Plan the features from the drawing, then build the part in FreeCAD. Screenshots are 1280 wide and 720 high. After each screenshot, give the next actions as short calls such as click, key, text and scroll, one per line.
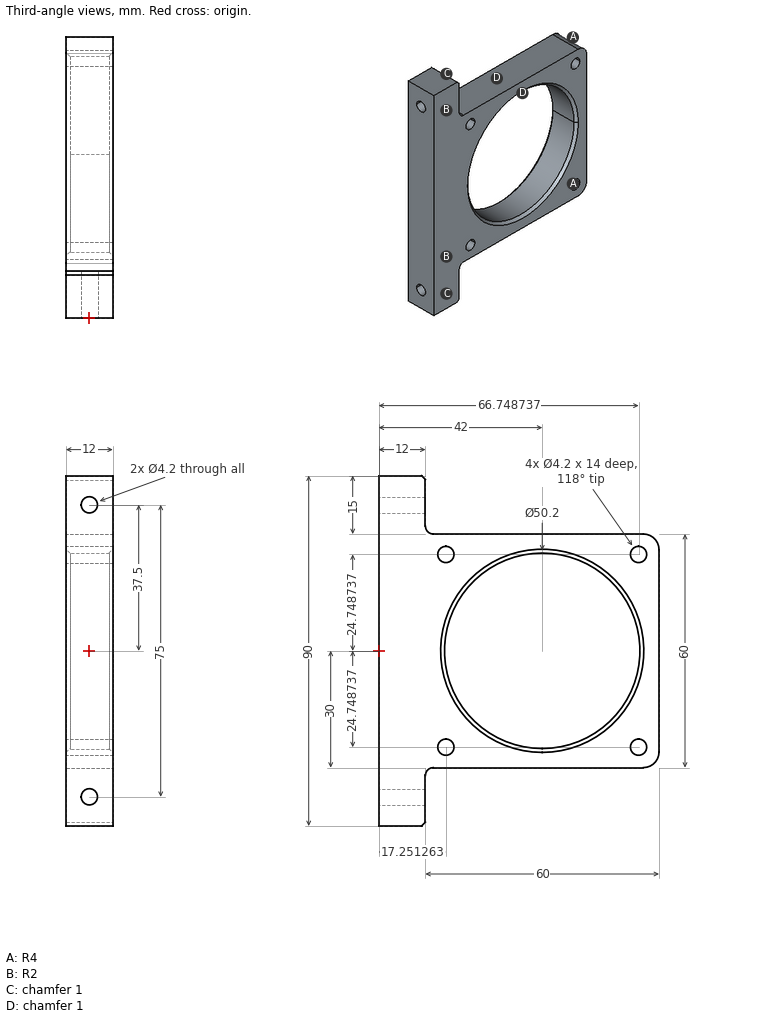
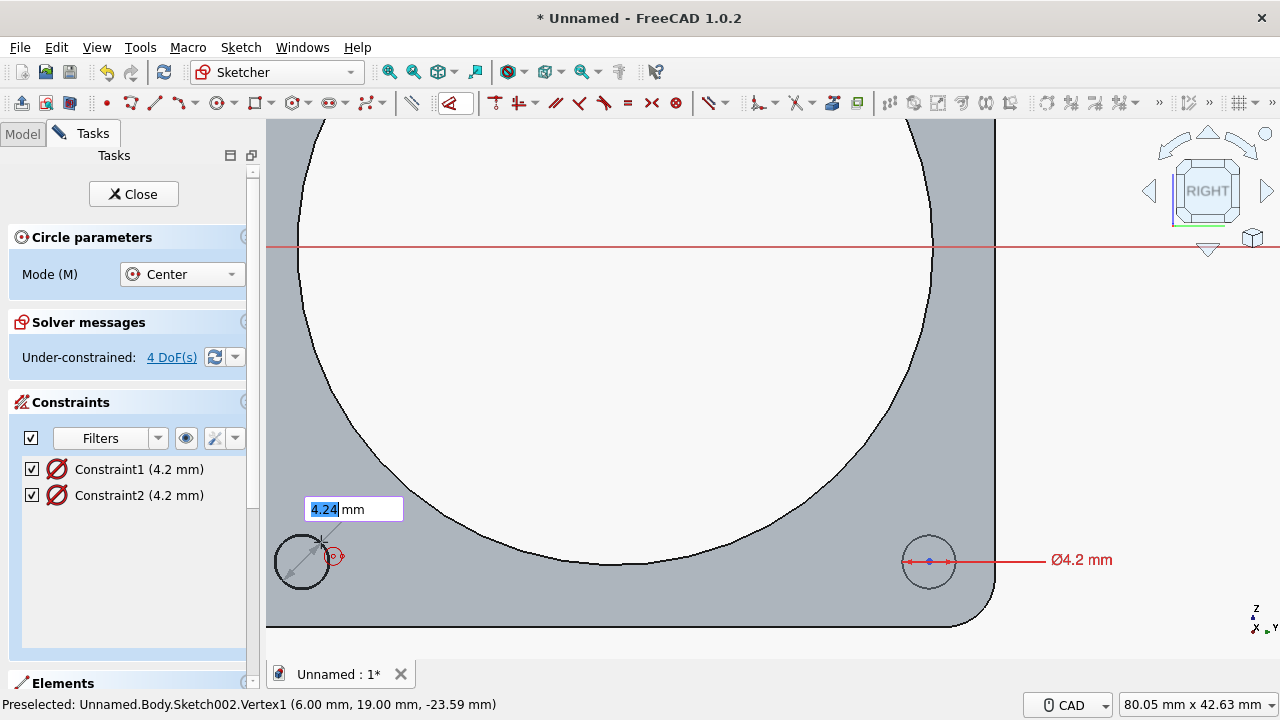
text(4.2)
key(Return)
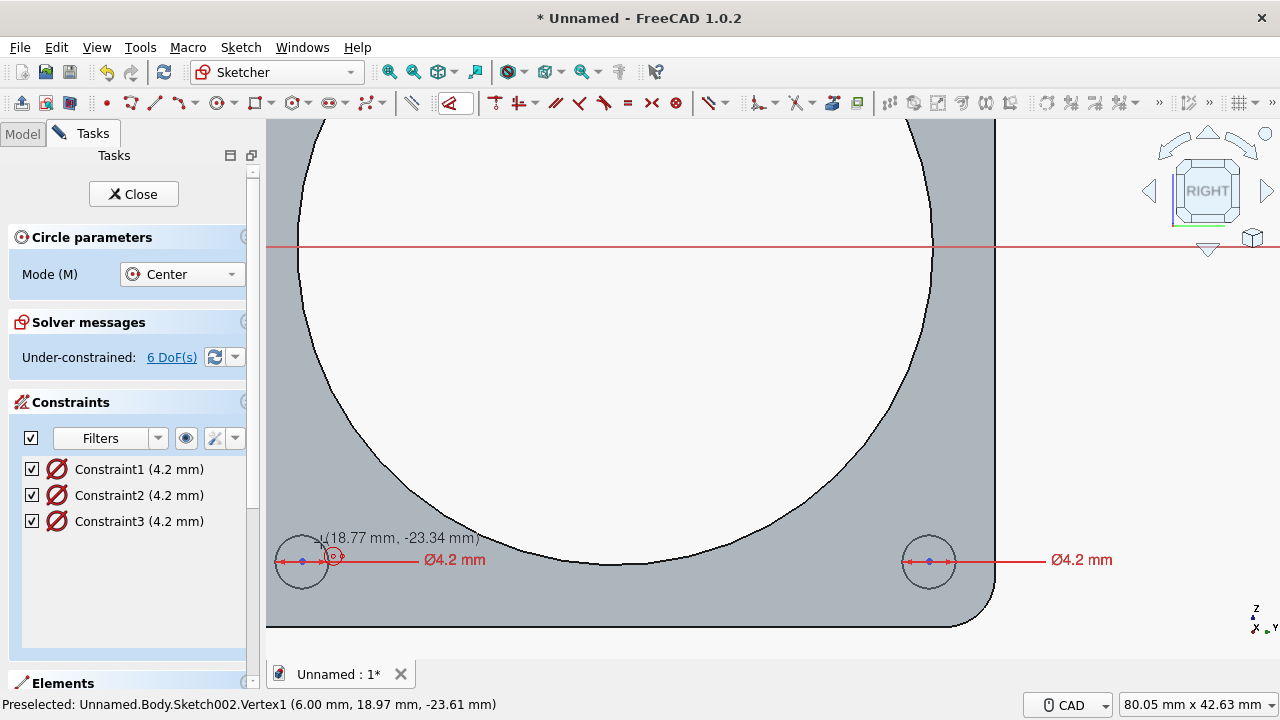
scroll(930, 561, down, 3)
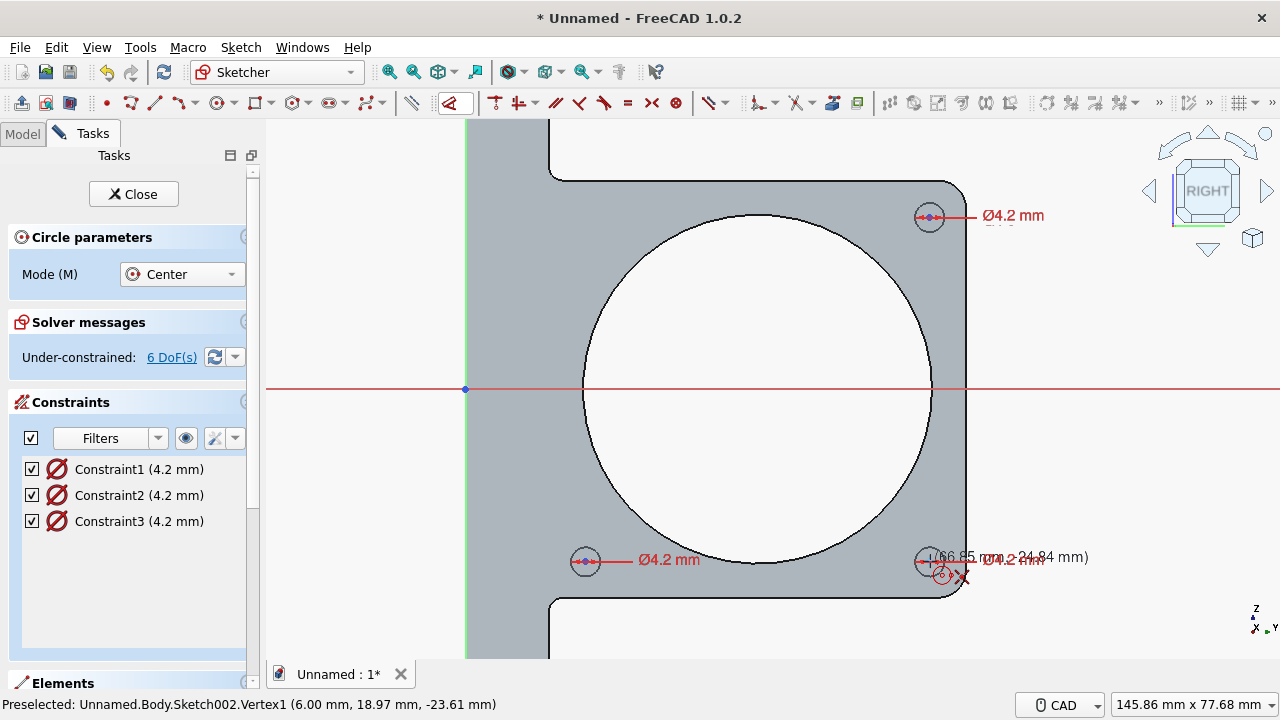
scroll(585, 217, up, 3)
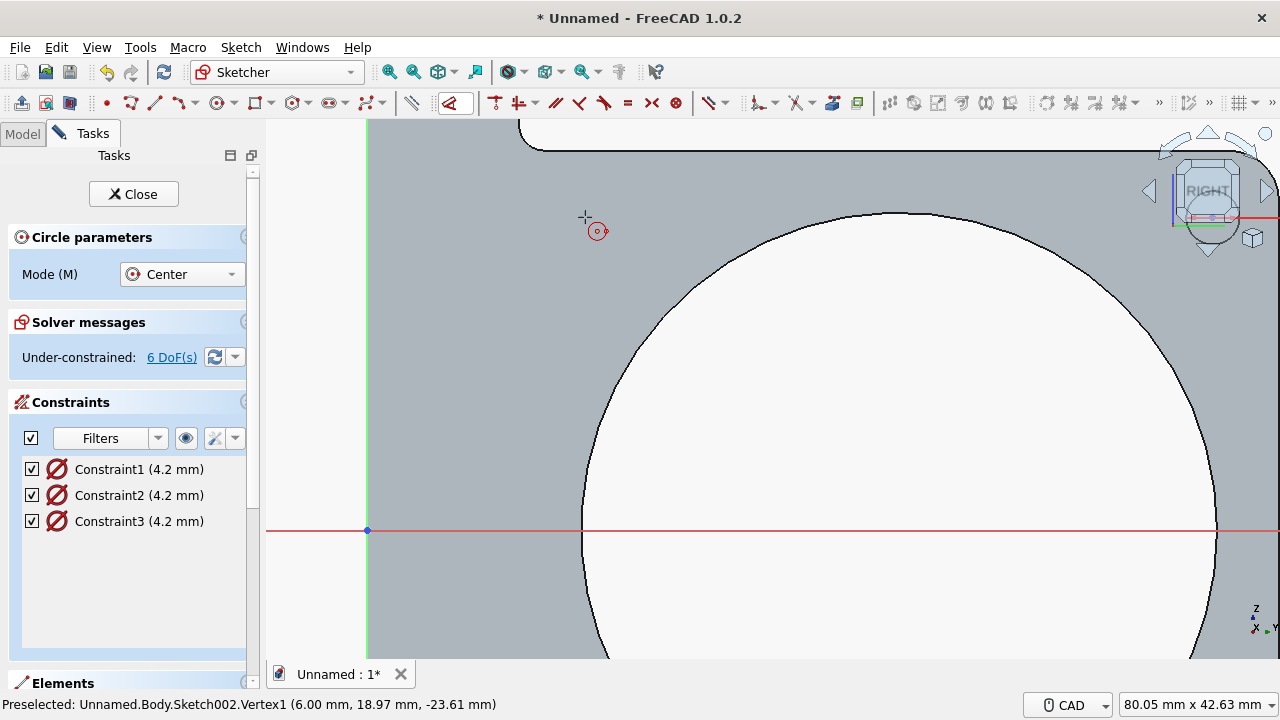
click(586, 217)
move(604, 198)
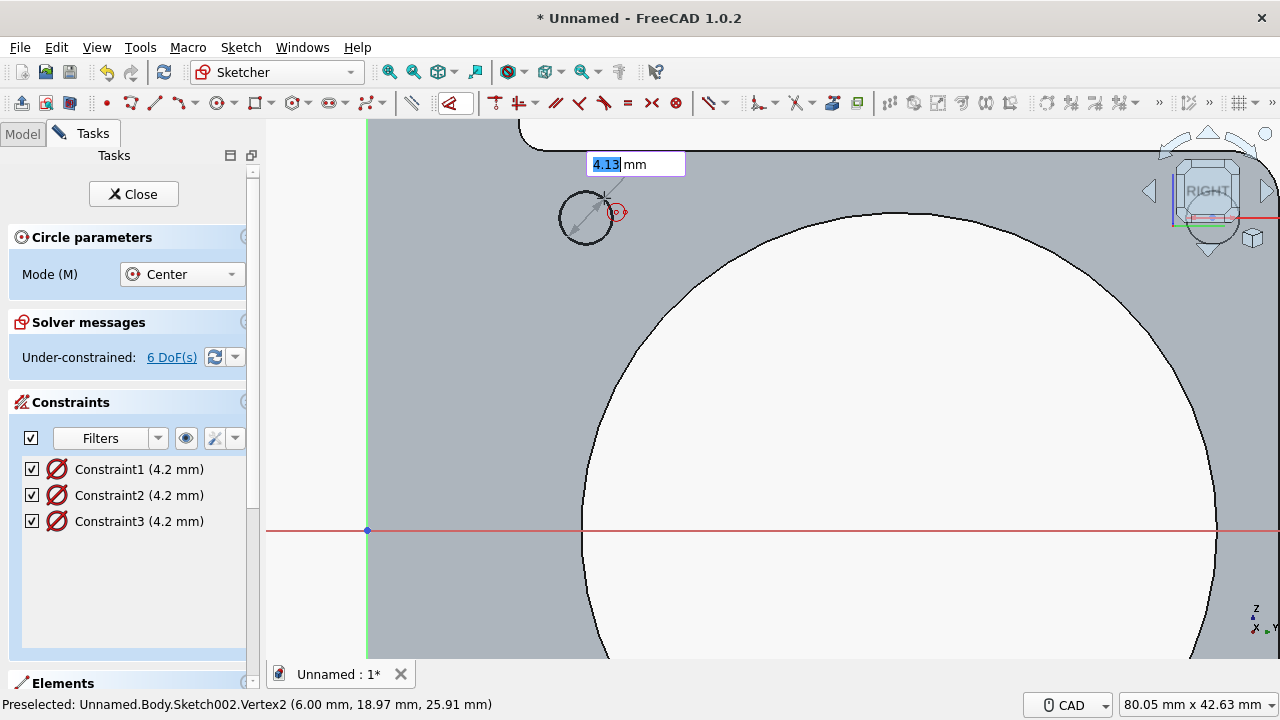
text(4.2)
key(Return)
key(Escape)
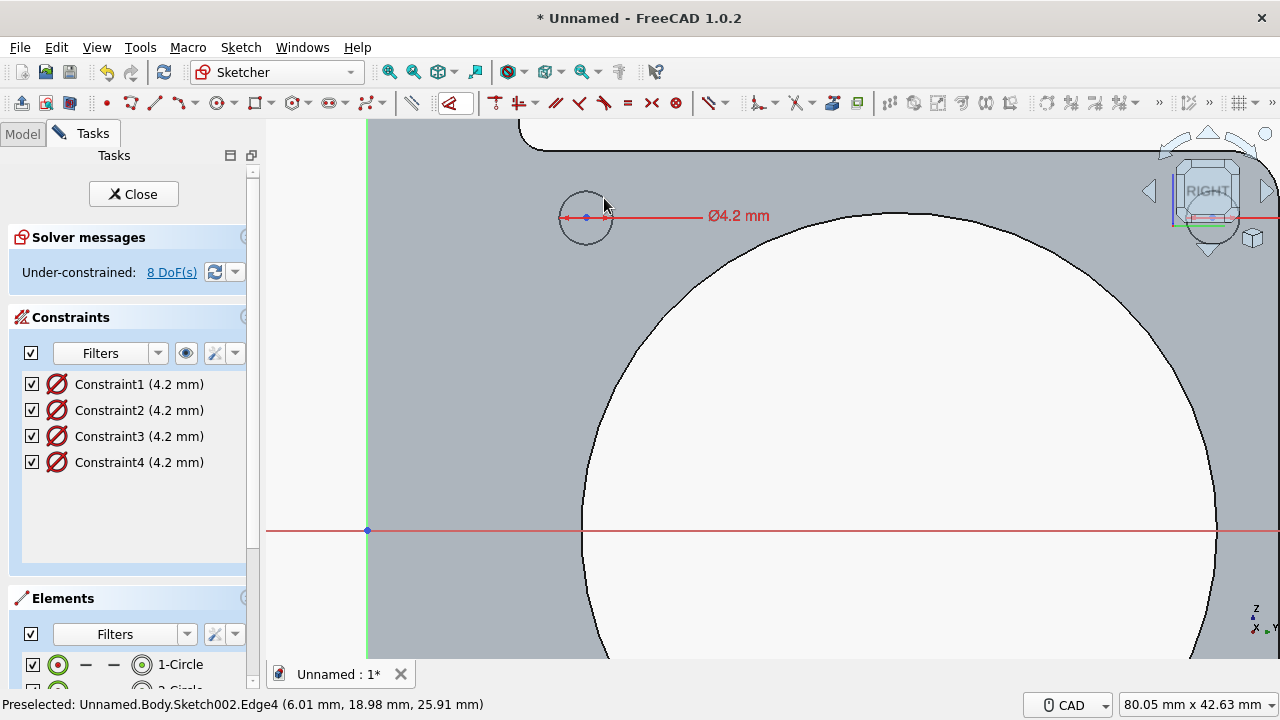
scroll(585, 217, down, 3)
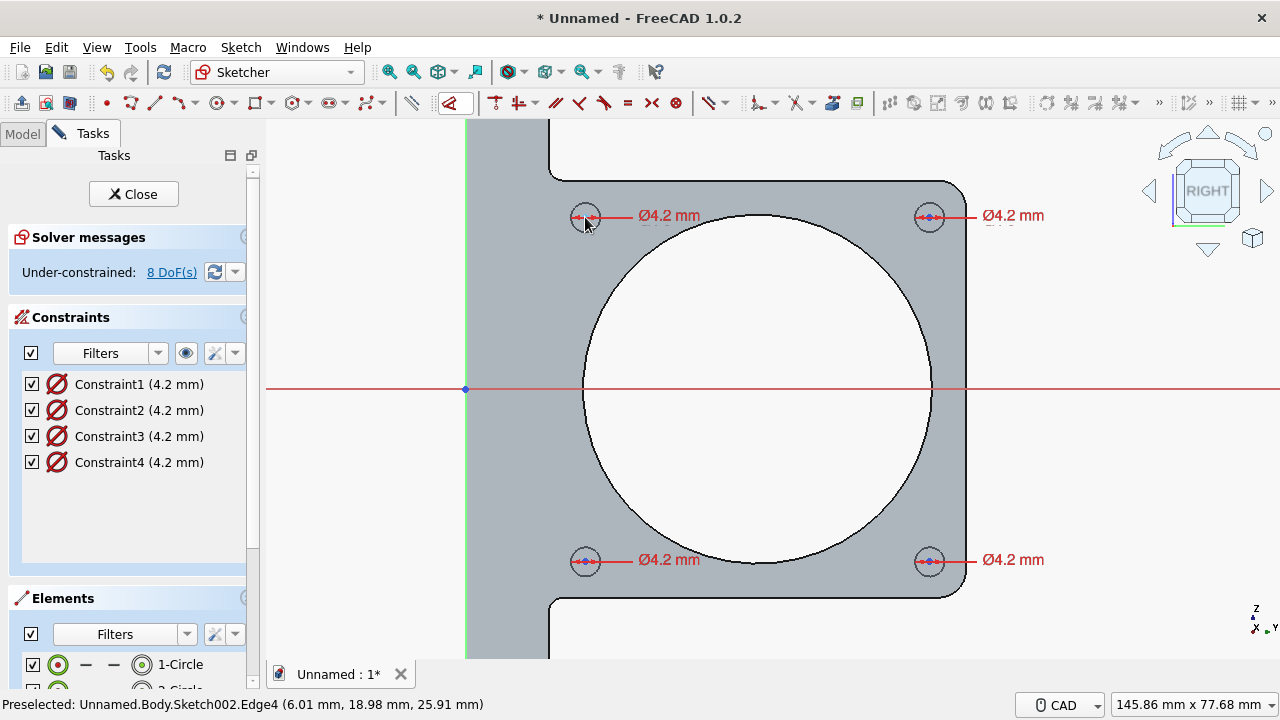
click(930, 218)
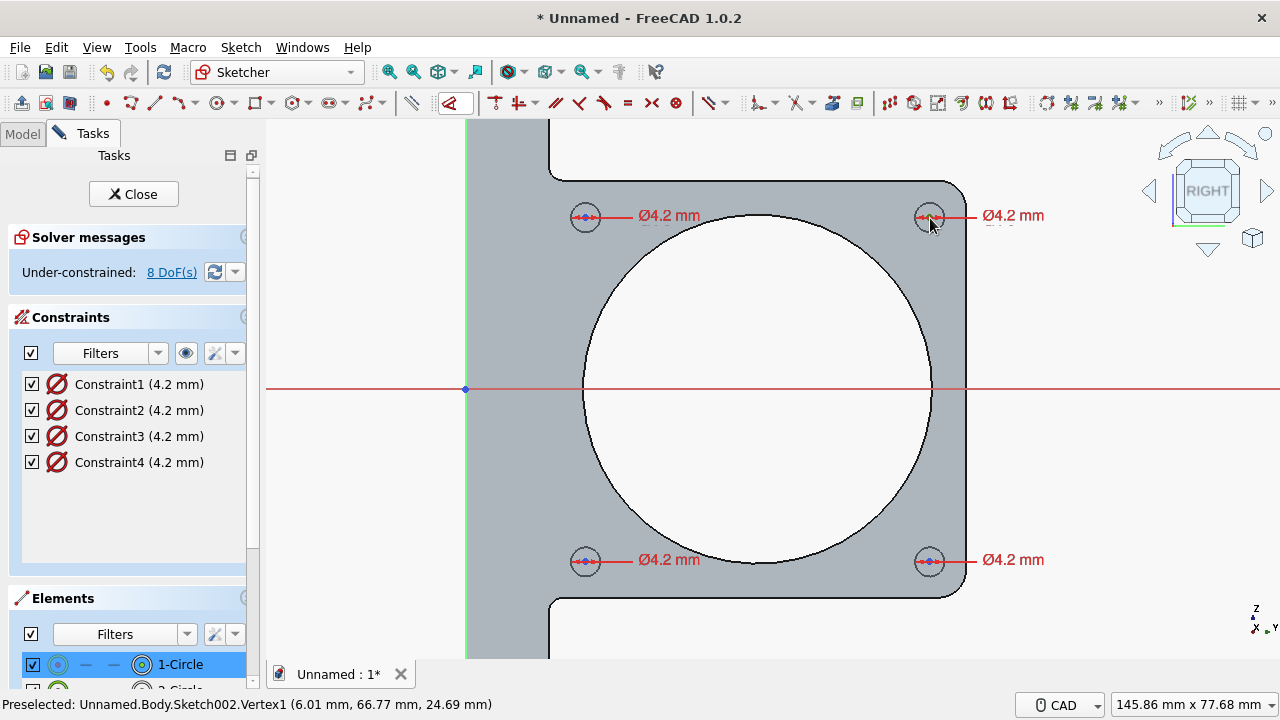
click(930, 562)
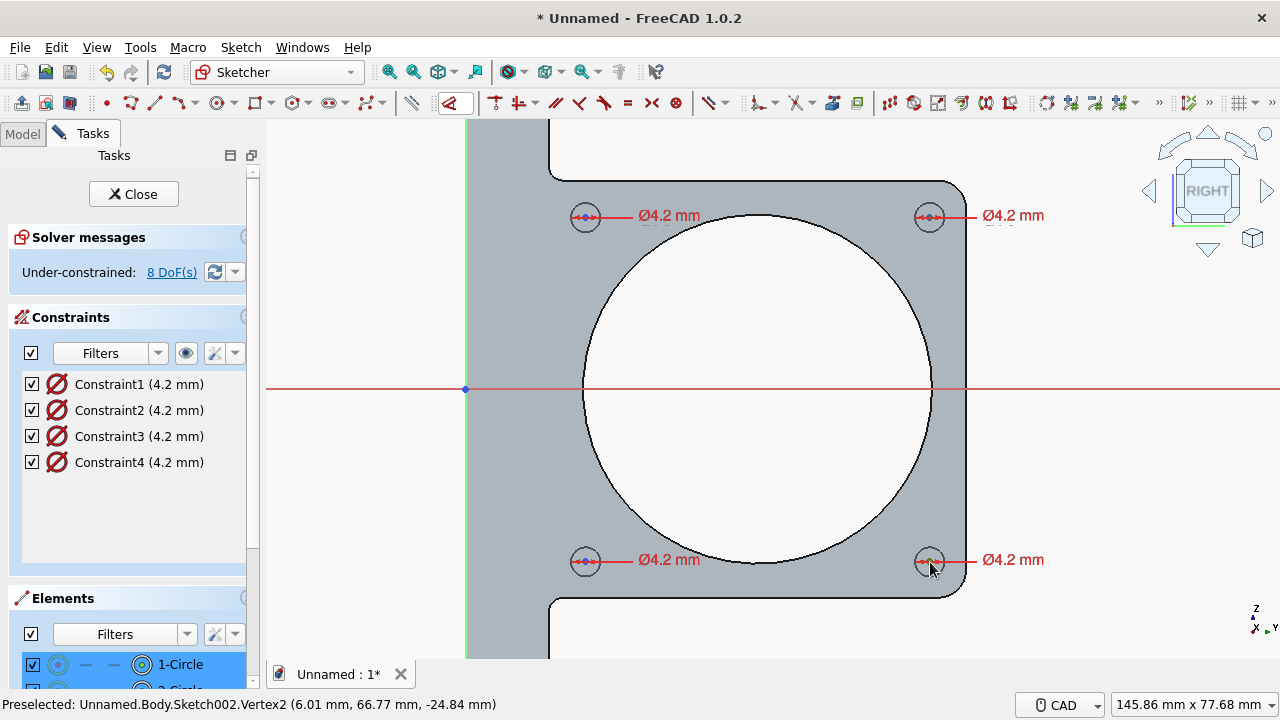
key(v)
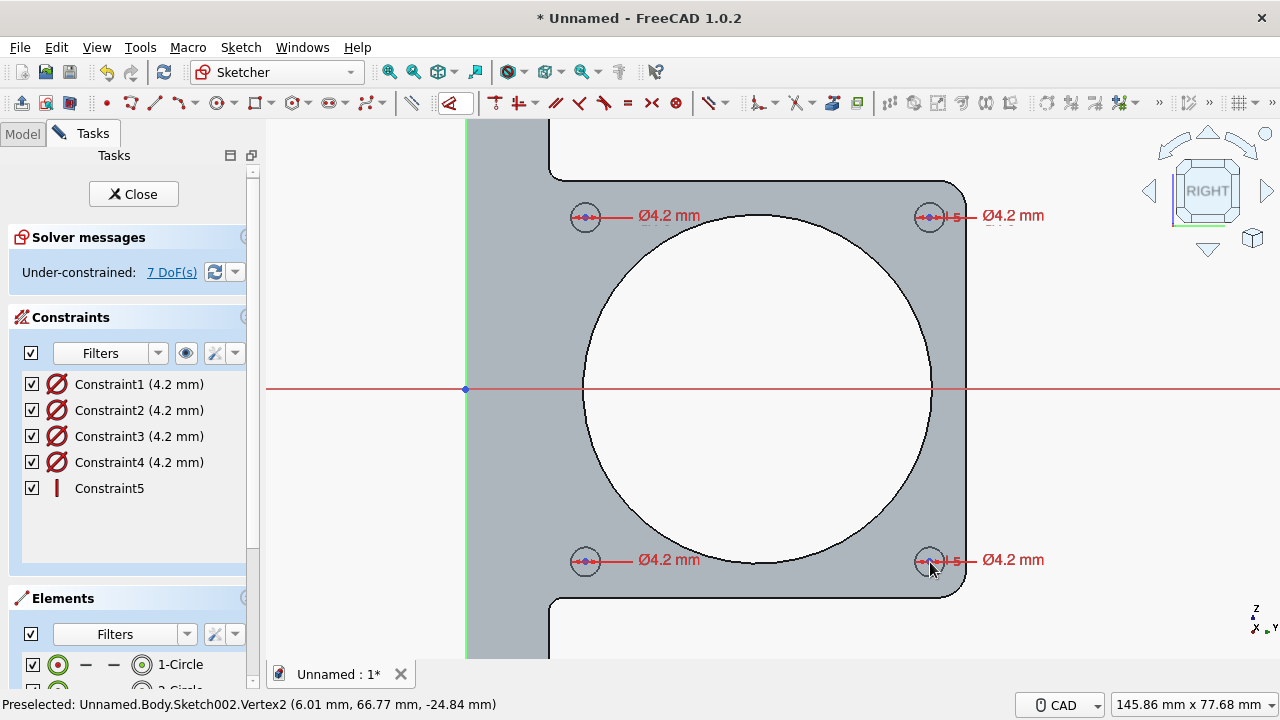
click(930, 562)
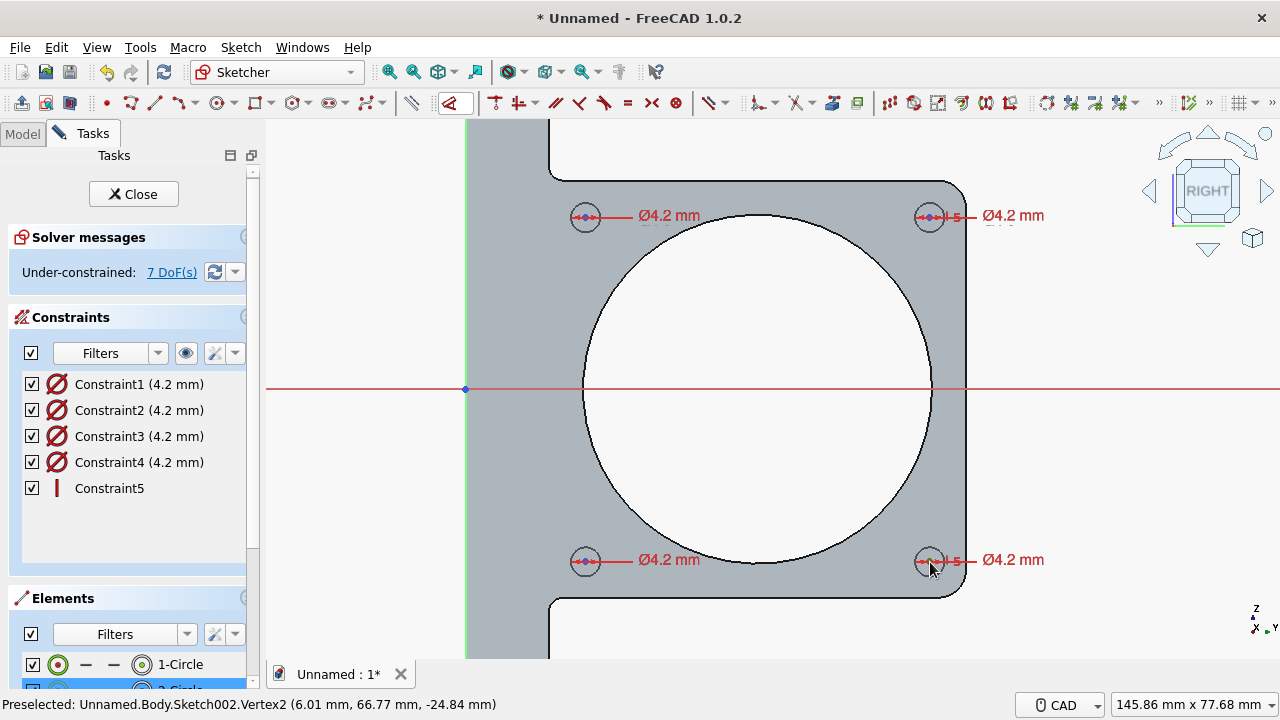
click(586, 562)